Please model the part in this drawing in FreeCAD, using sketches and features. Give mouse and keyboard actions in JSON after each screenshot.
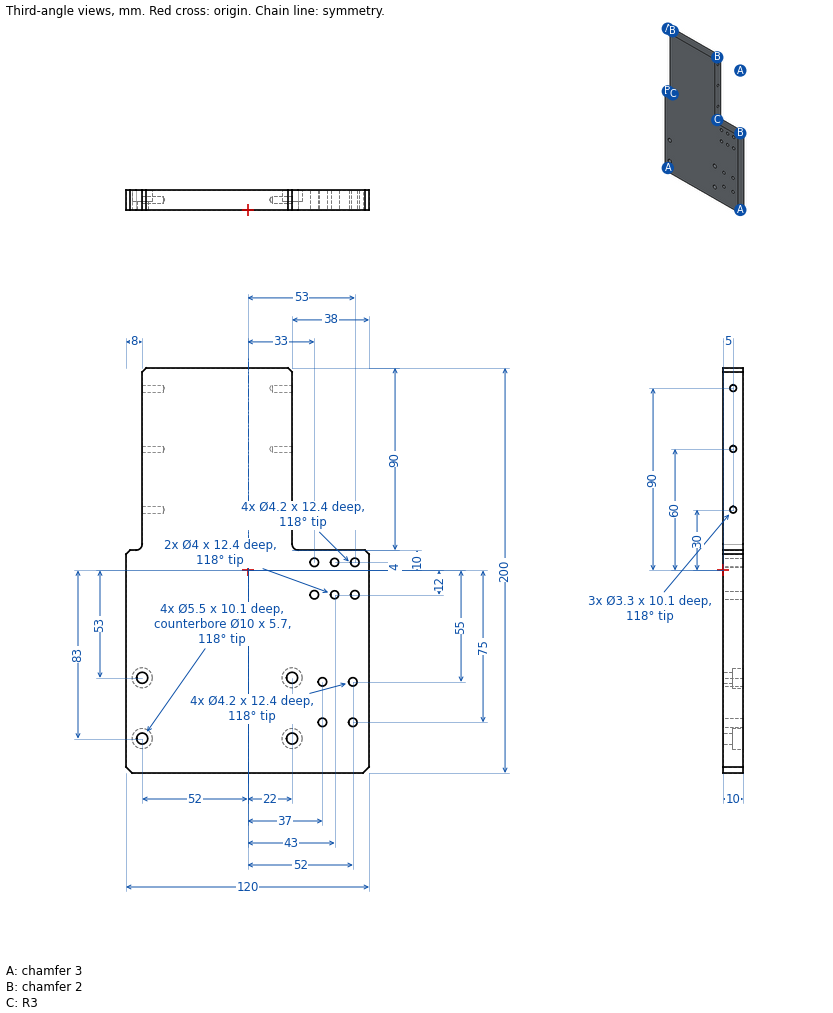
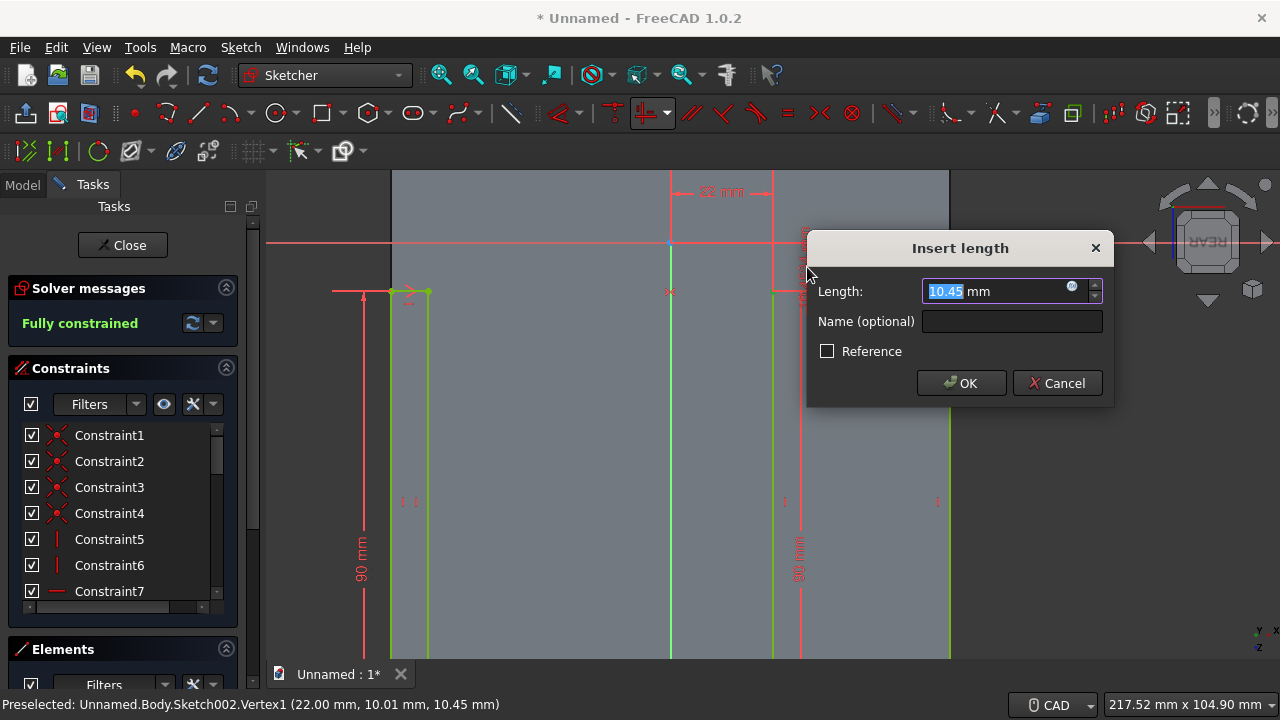
{"action": "type", "text": "10"}
{"action": "key", "text": "Return"}
{"action": "key", "text": "Escape"}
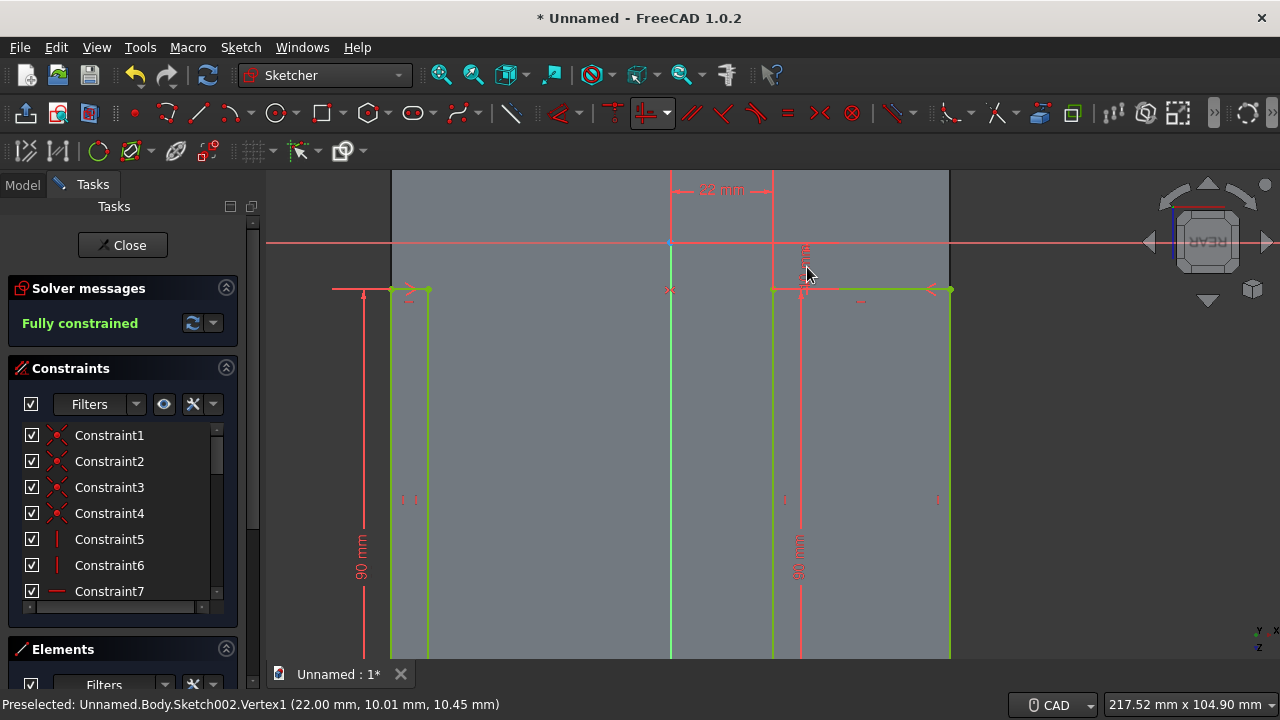
{"action": "left_click", "coordinate": [123, 245]}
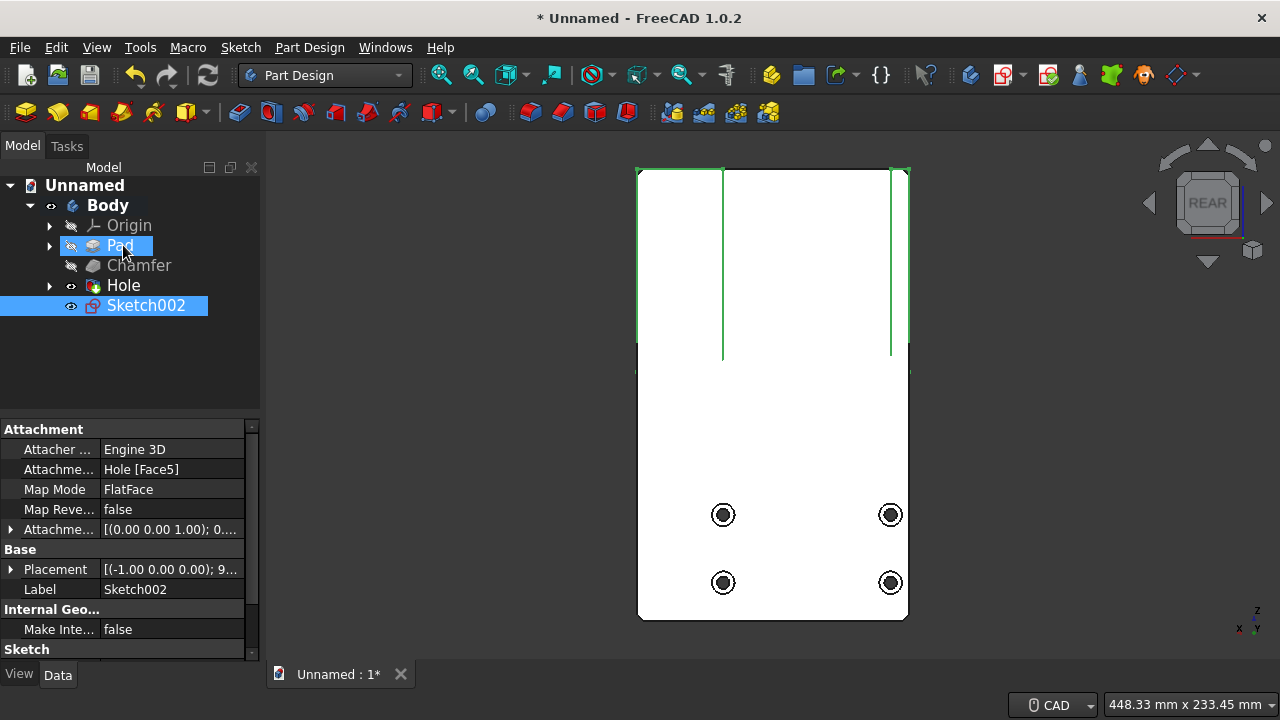
{"action": "left_click", "coordinate": [240, 112]}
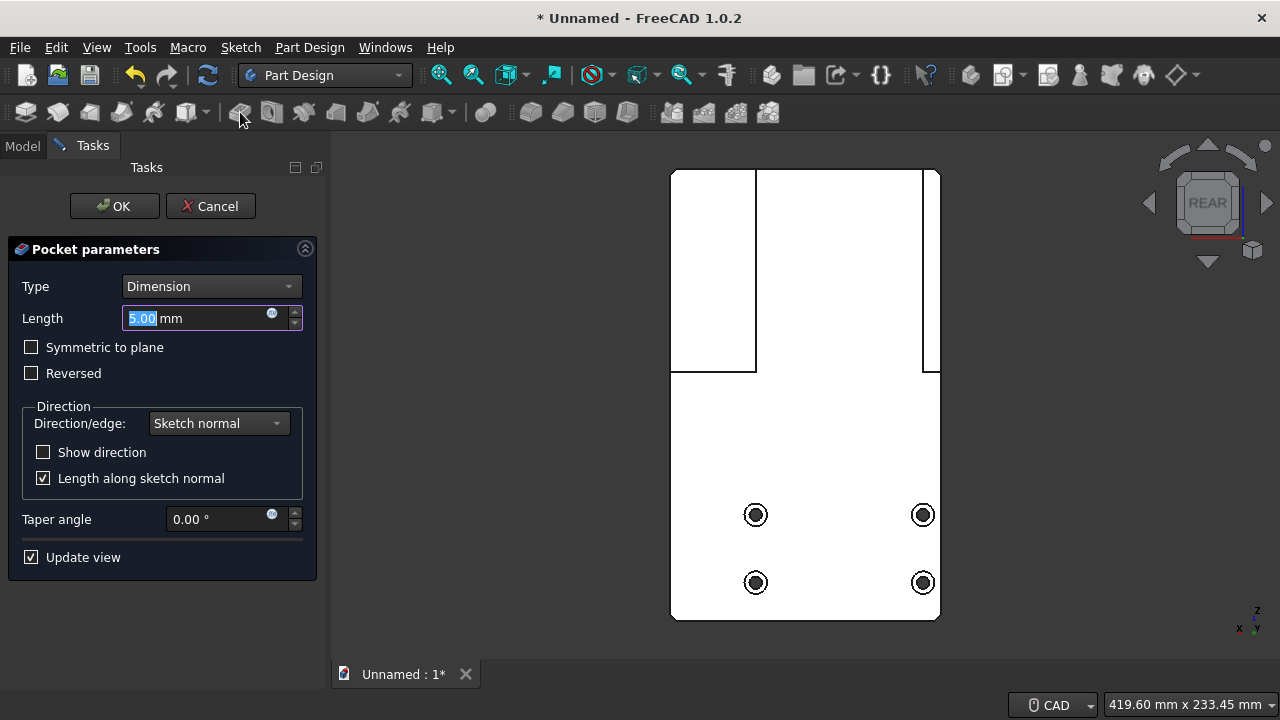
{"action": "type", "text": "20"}
{"action": "key", "text": "Tab"}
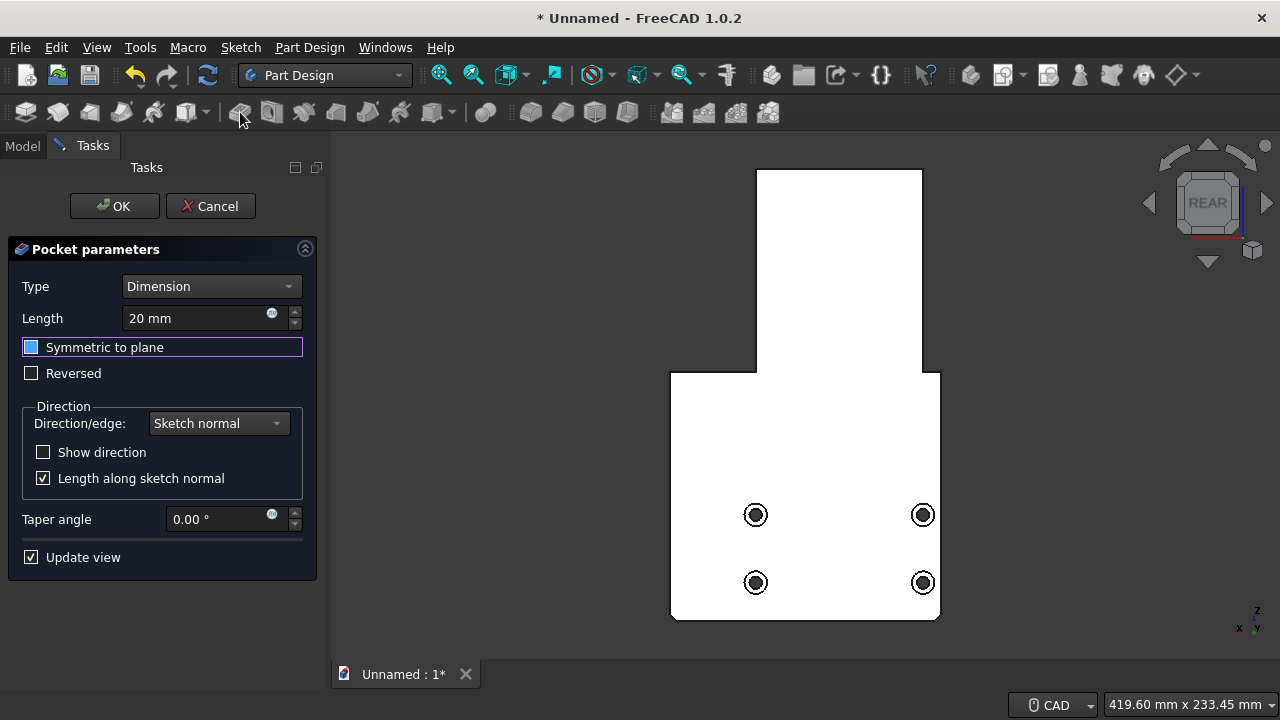
{"action": "left_click", "coordinate": [115, 206]}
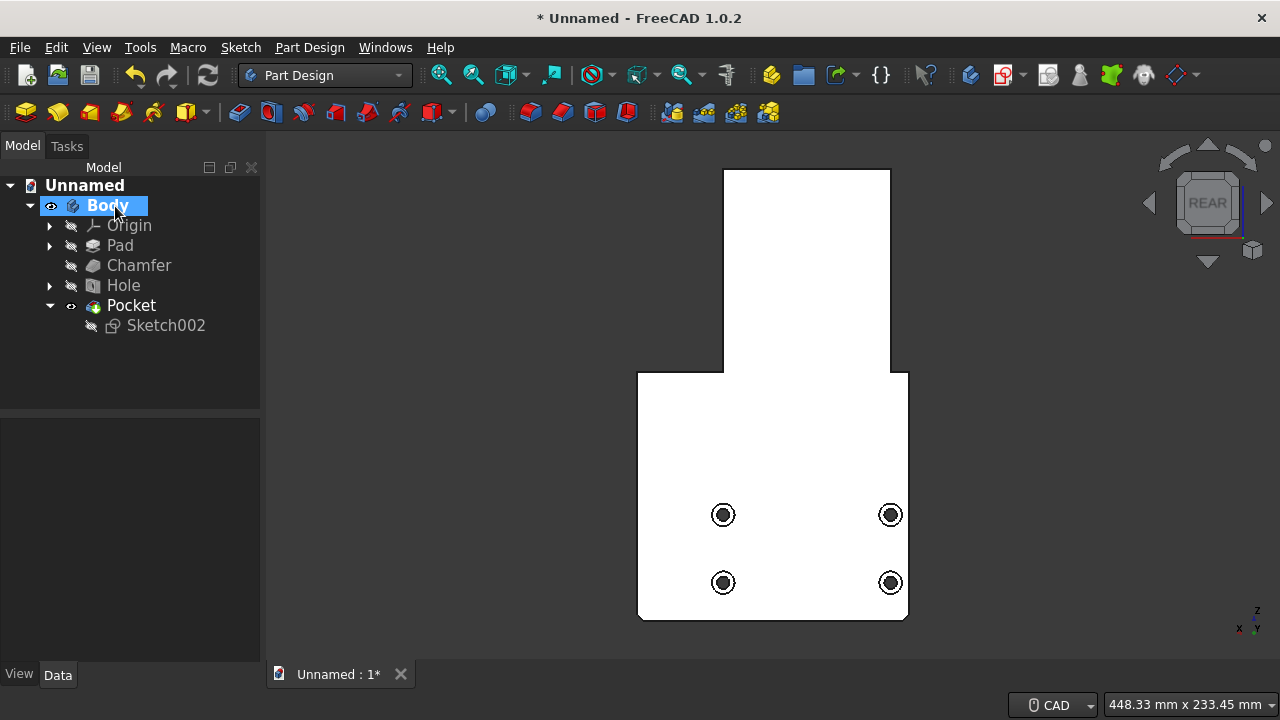
{"action": "key", "text": "0"}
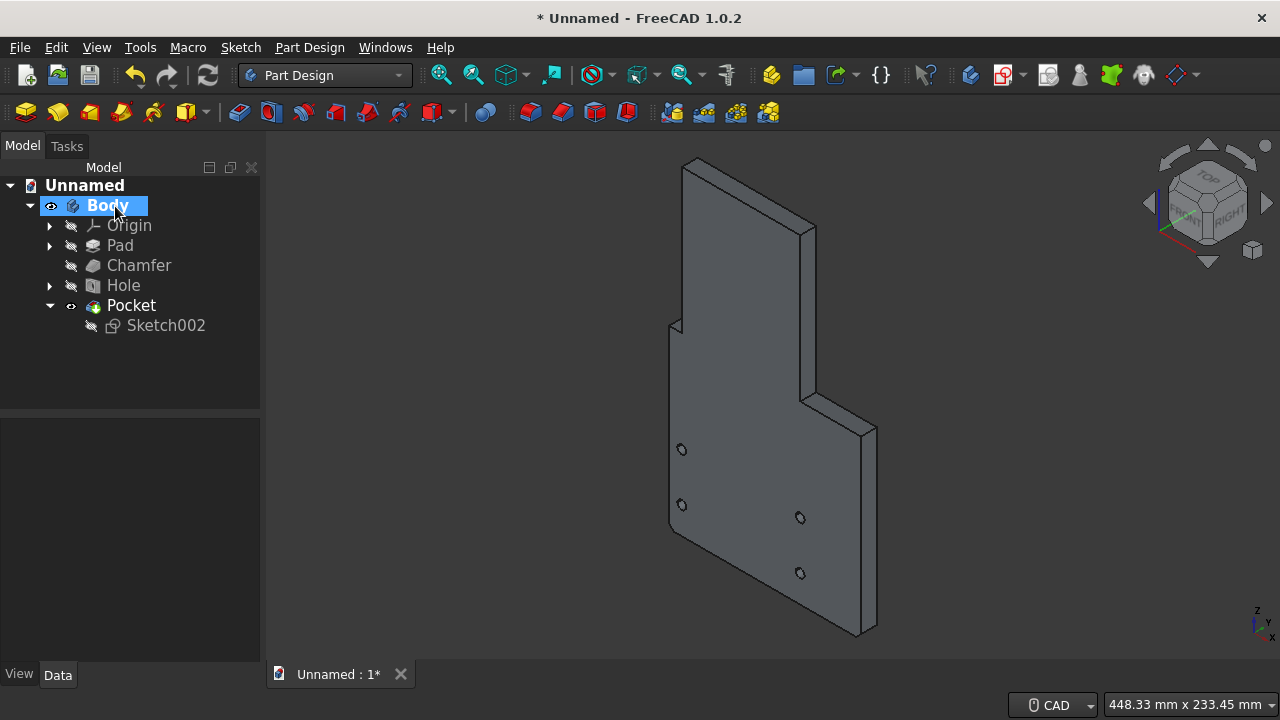
{"action": "left_click", "coordinate": [808, 230]}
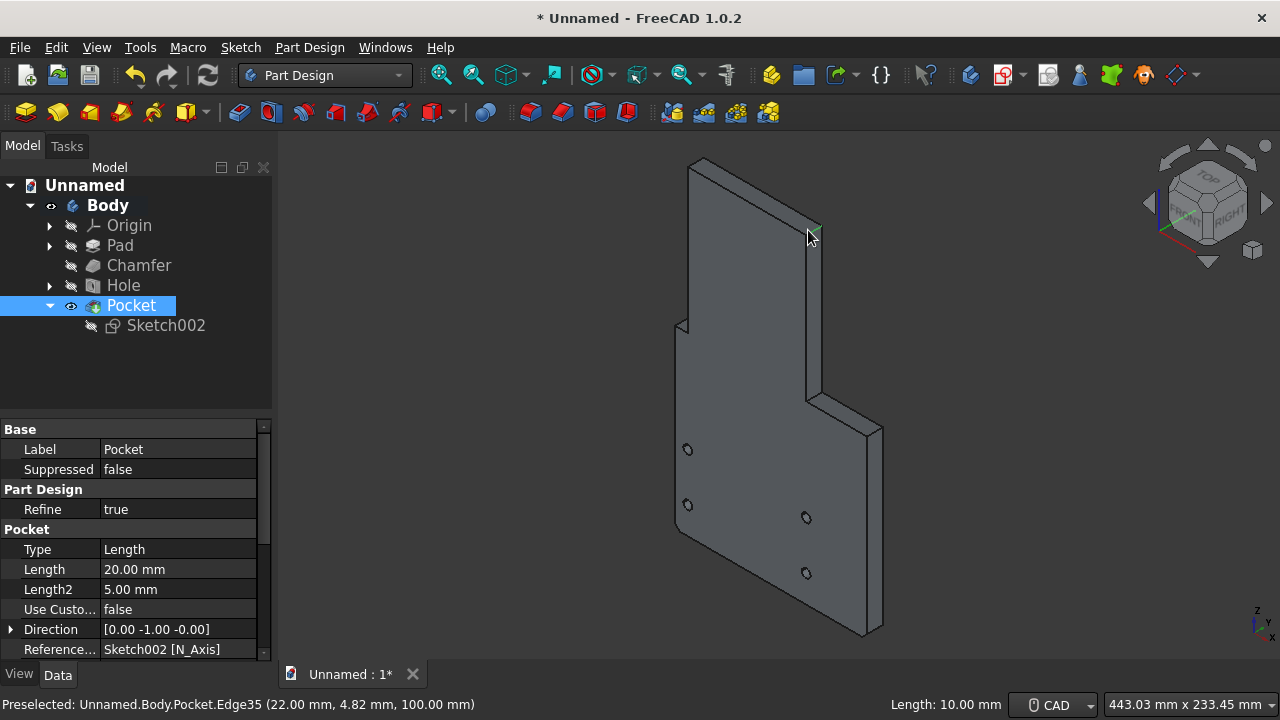
{"action": "left_click", "coordinate": [875, 431], "text": "ctrl"}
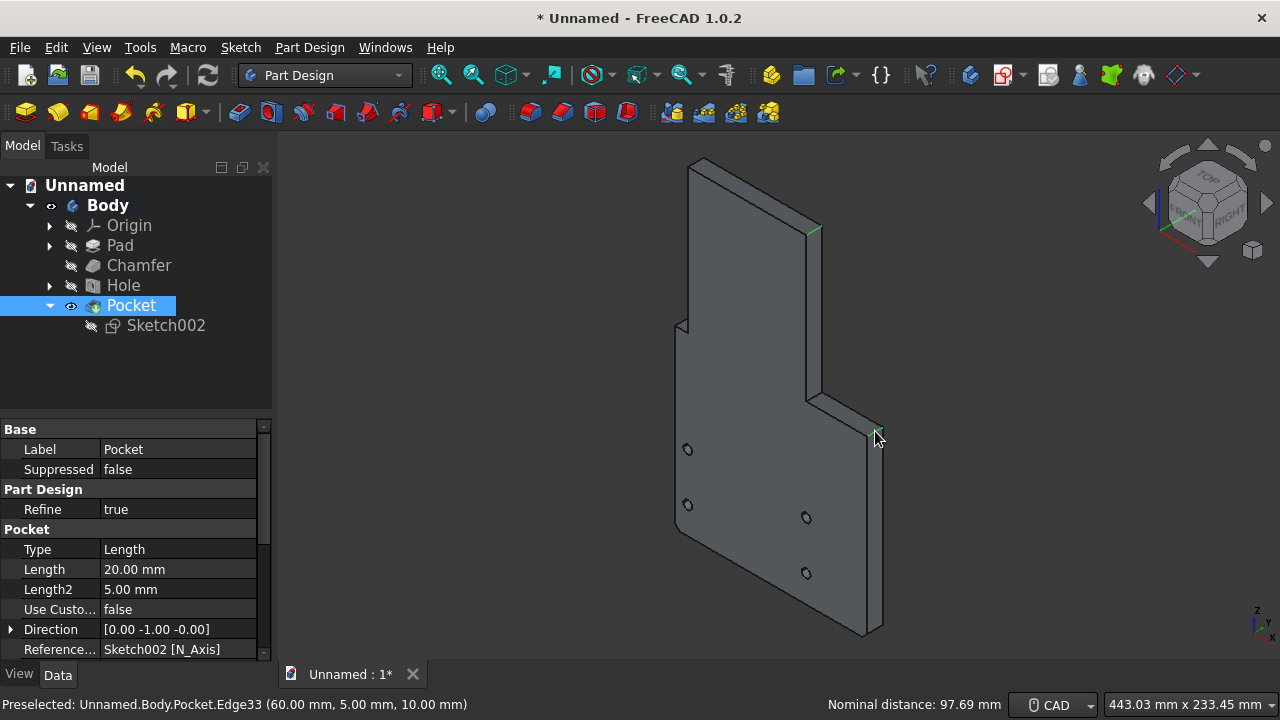
{"action": "key", "text": "2"}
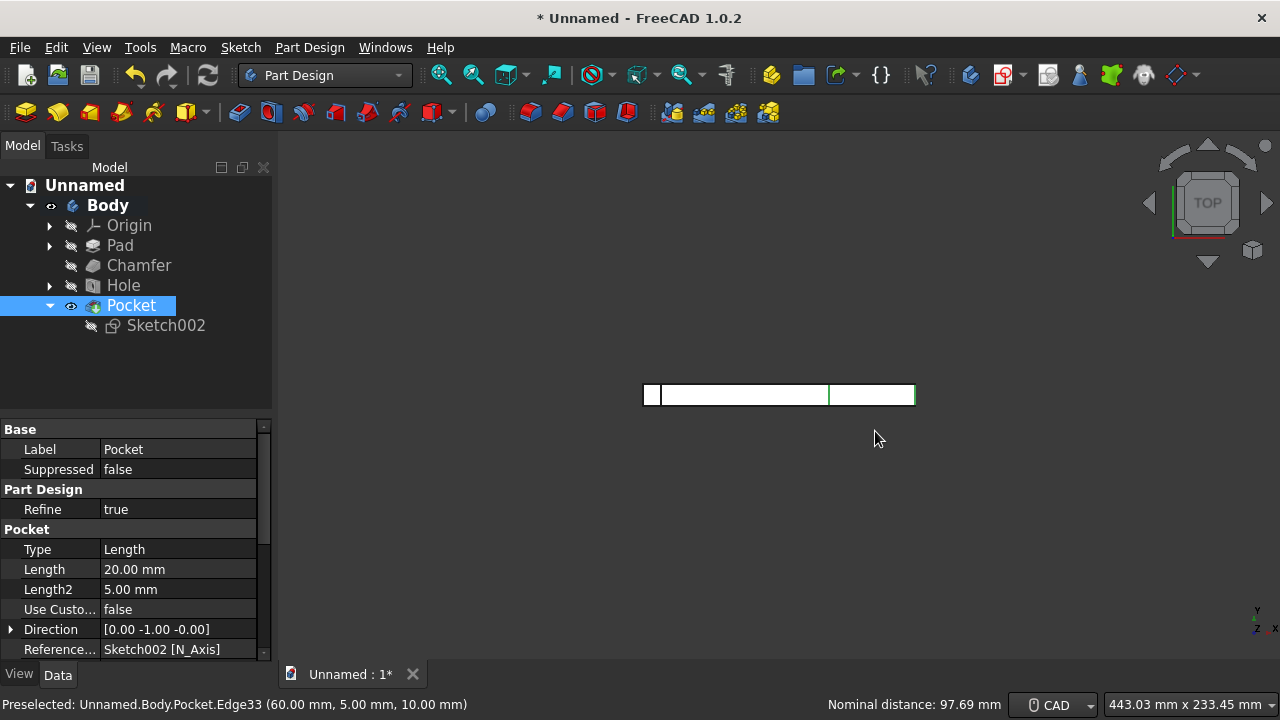
{"action": "left_click", "coordinate": [442, 76]}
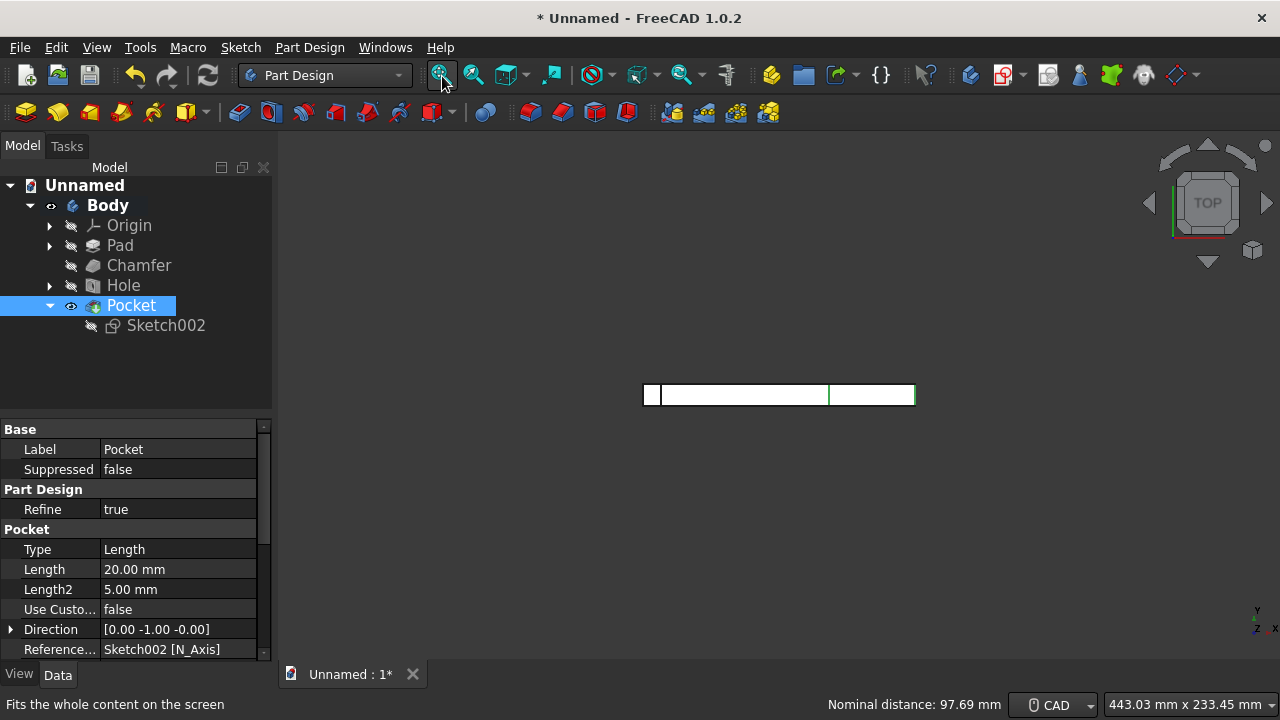
{"action": "left_click", "coordinate": [643, 394], "text": "ctrl"}